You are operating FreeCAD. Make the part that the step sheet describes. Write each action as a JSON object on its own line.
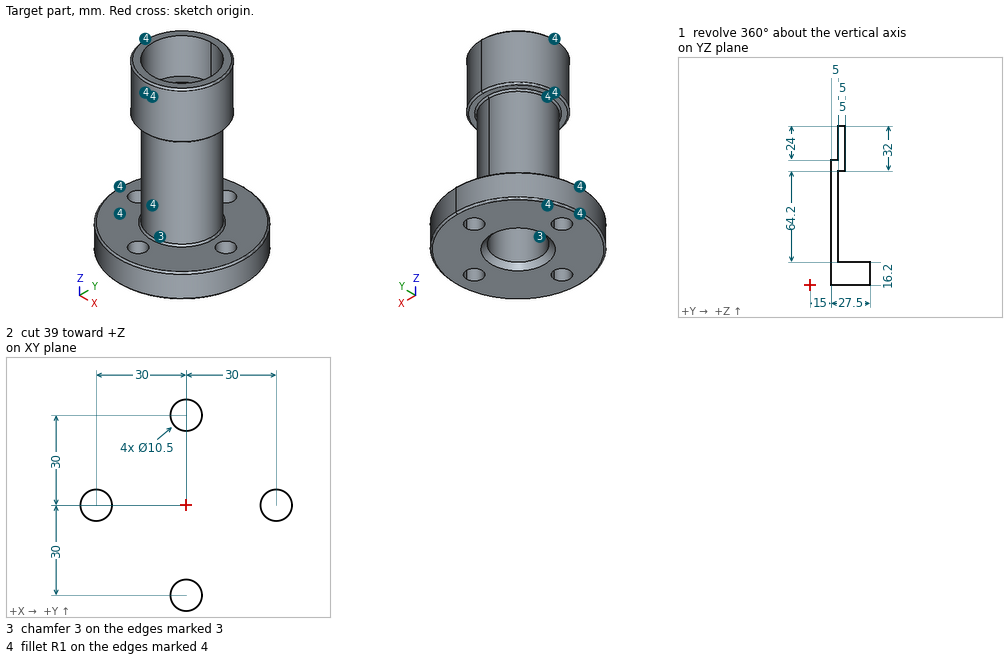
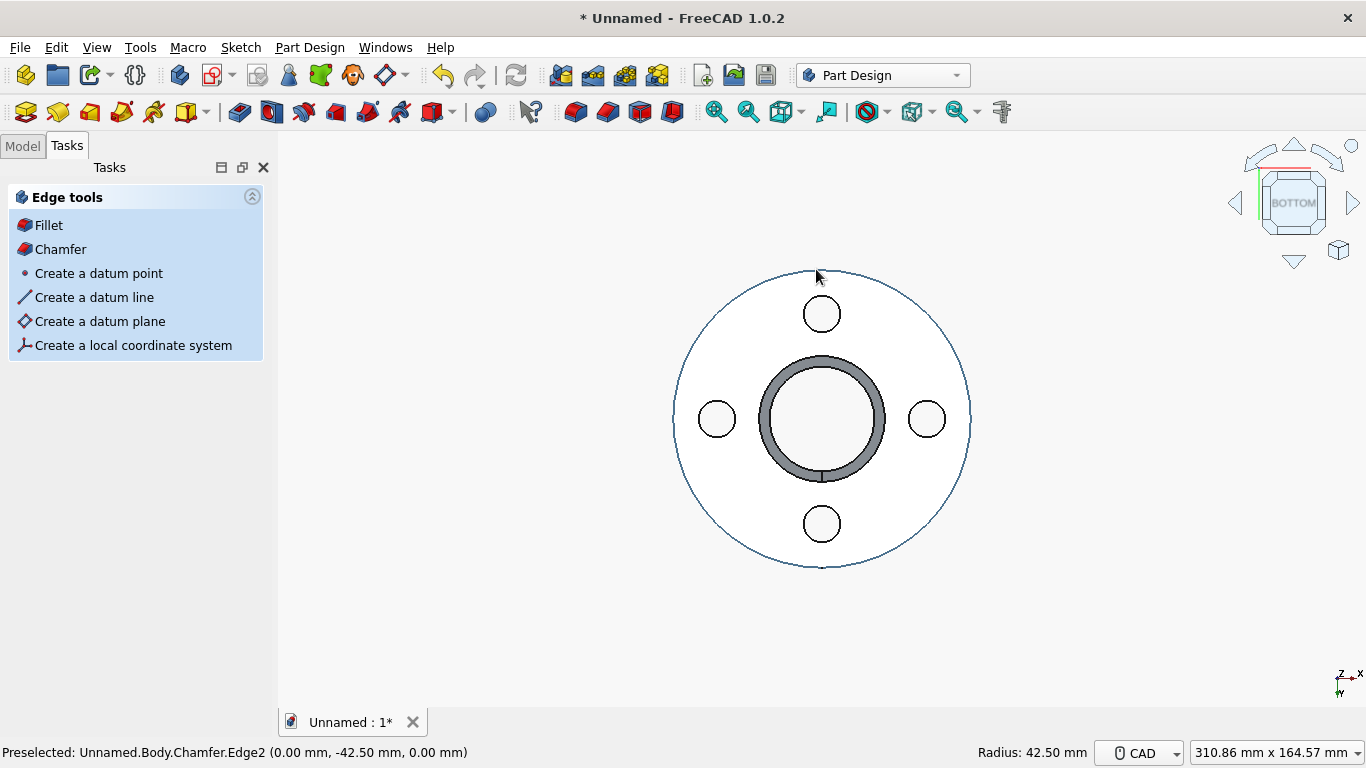
{"action": "key", "text": "0"}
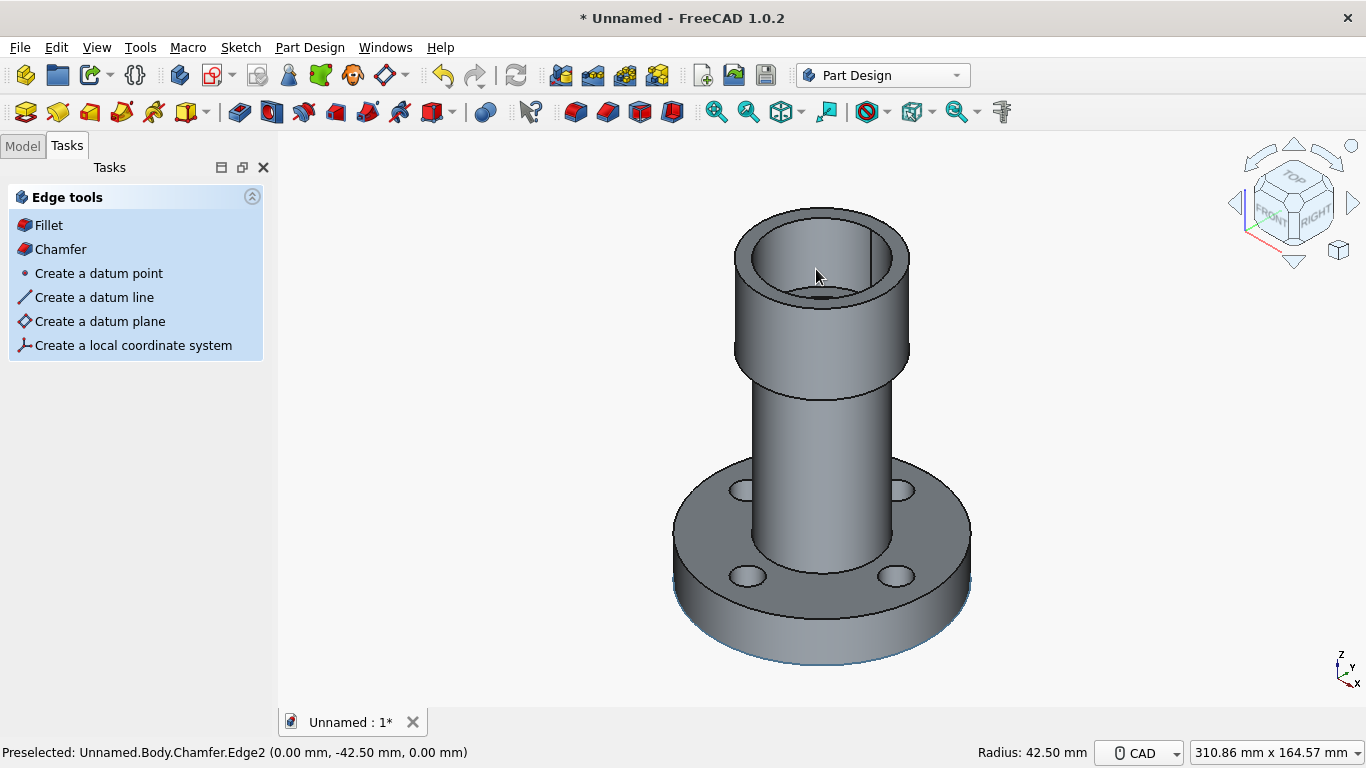
{"action": "left_click", "coordinate": [717, 593], "text": "ctrl"}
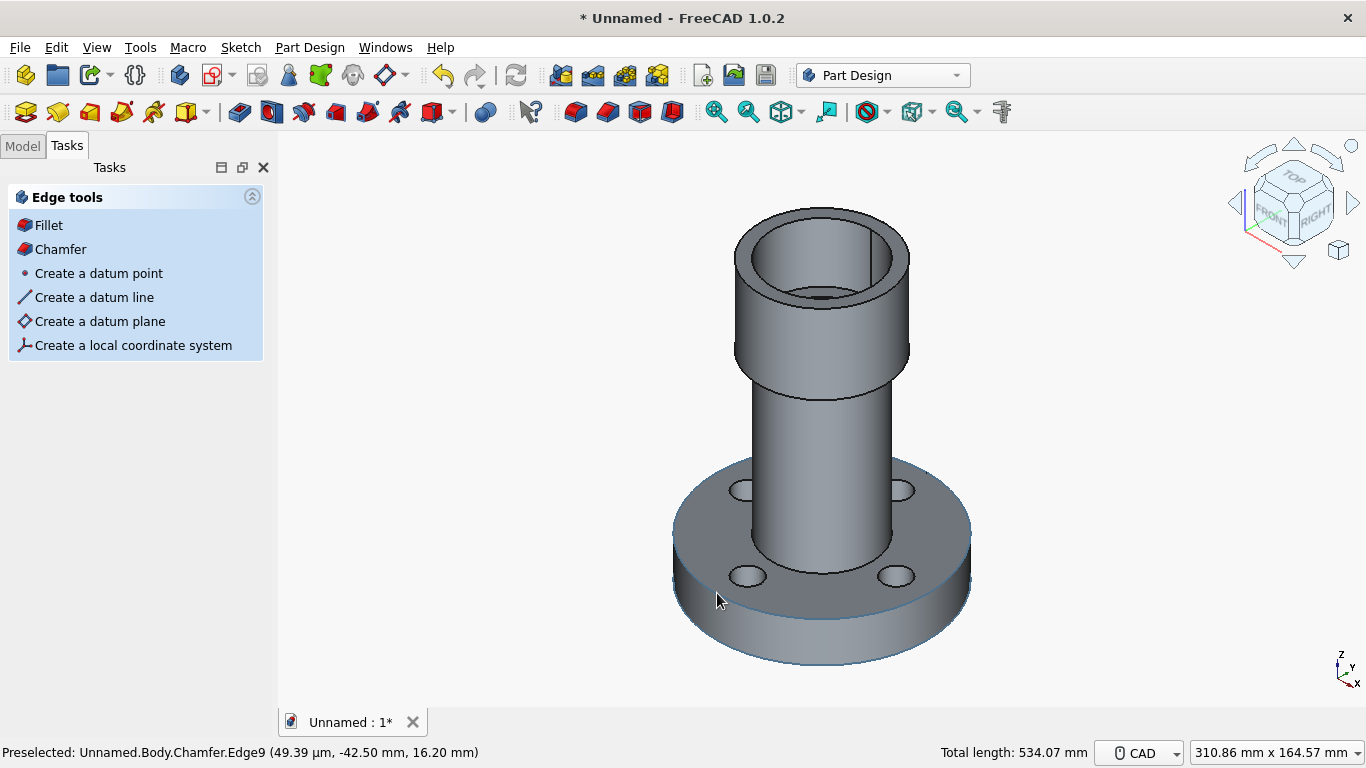
{"action": "left_click", "coordinate": [760, 293], "text": "ctrl"}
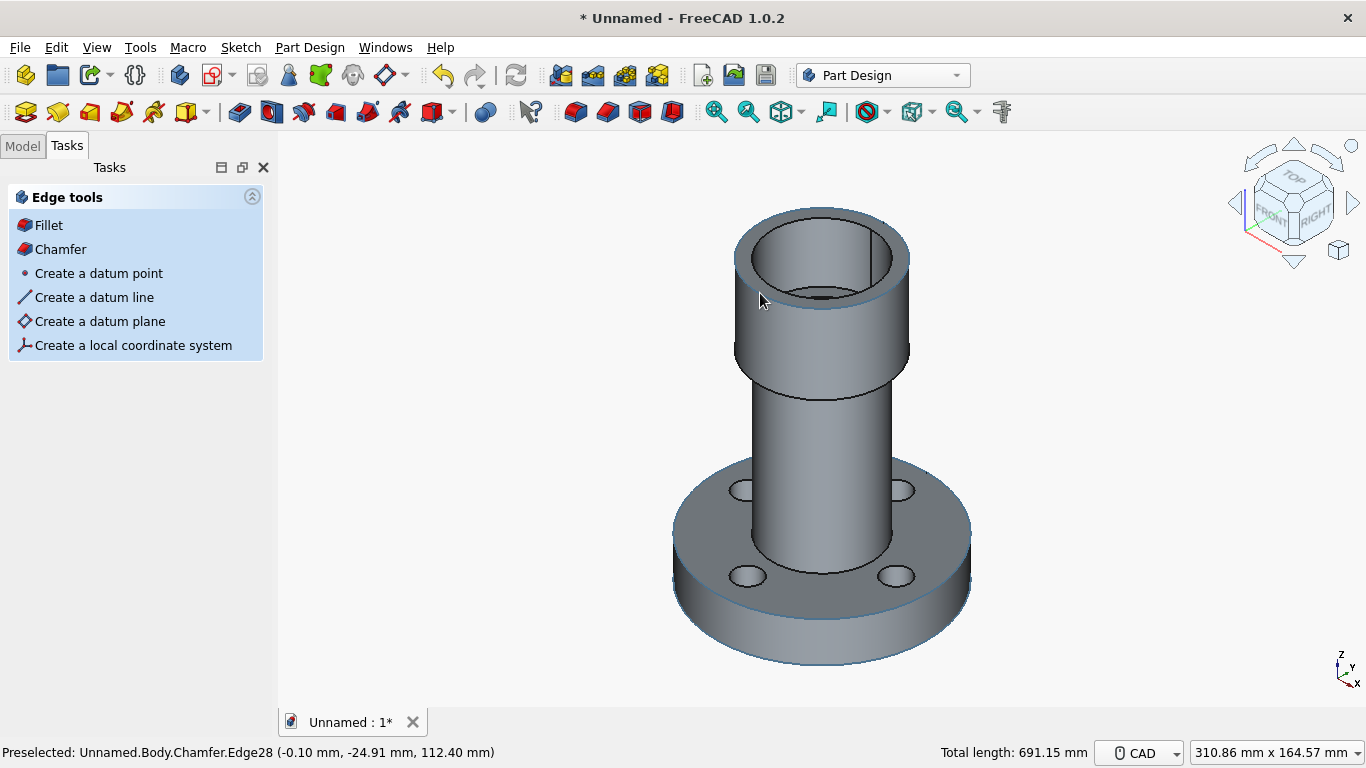
{"action": "key", "text": "2"}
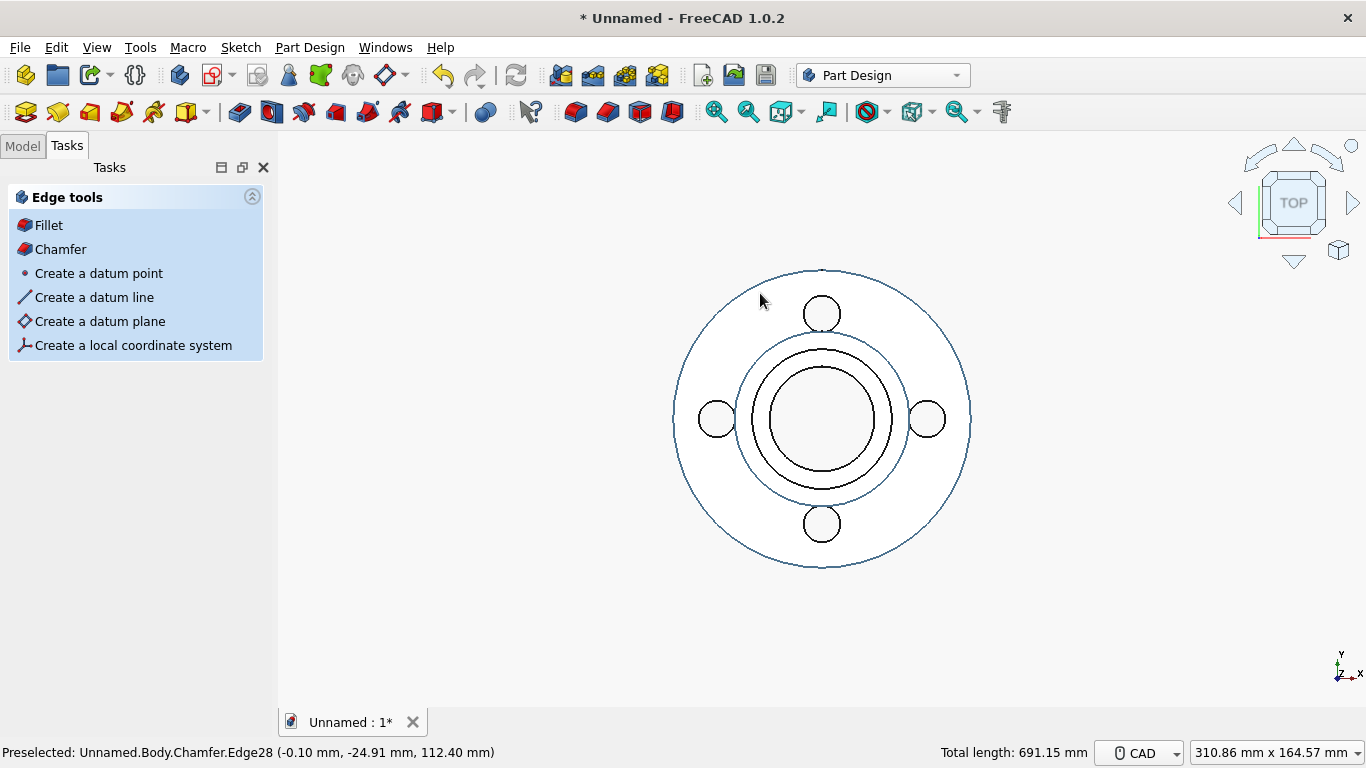
{"action": "key", "text": "1"}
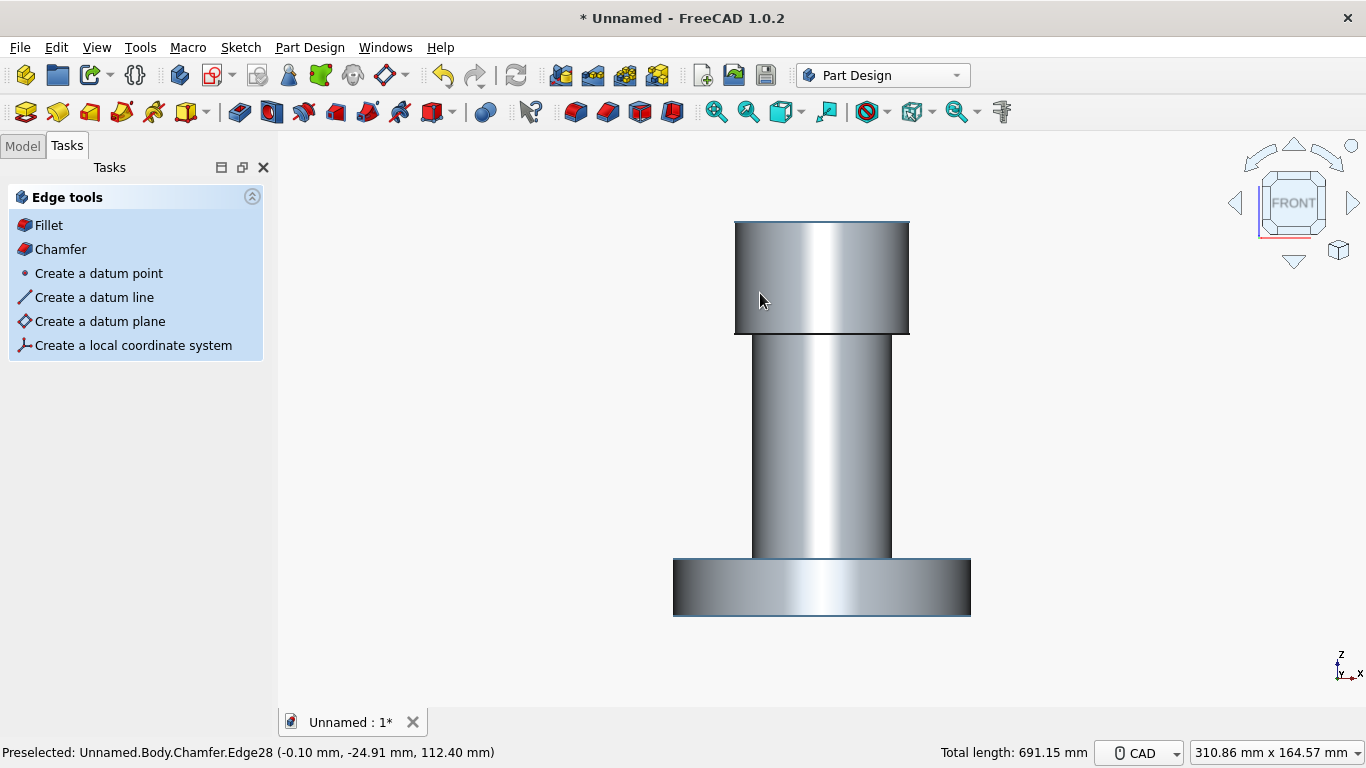
{"action": "left_click", "coordinate": [822, 333], "text": "ctrl"}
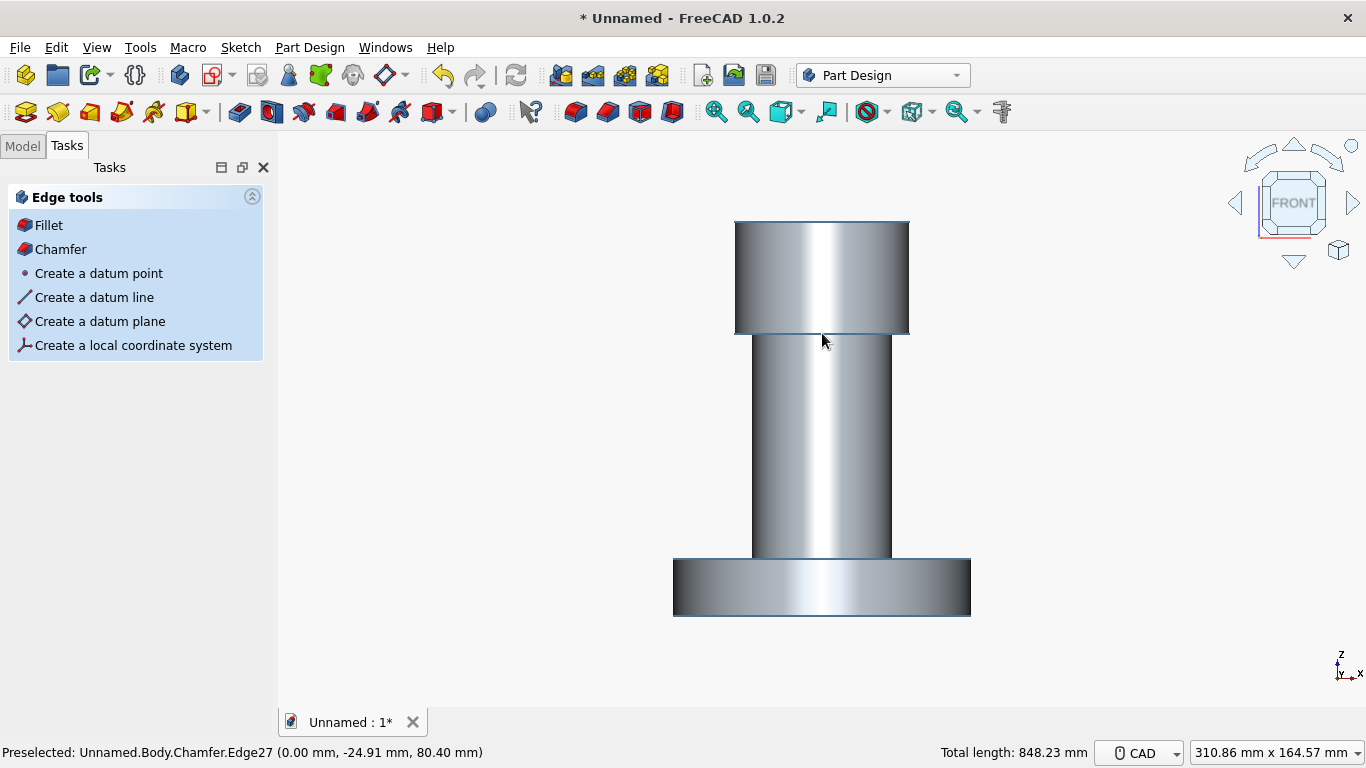
{"action": "key", "text": "3"}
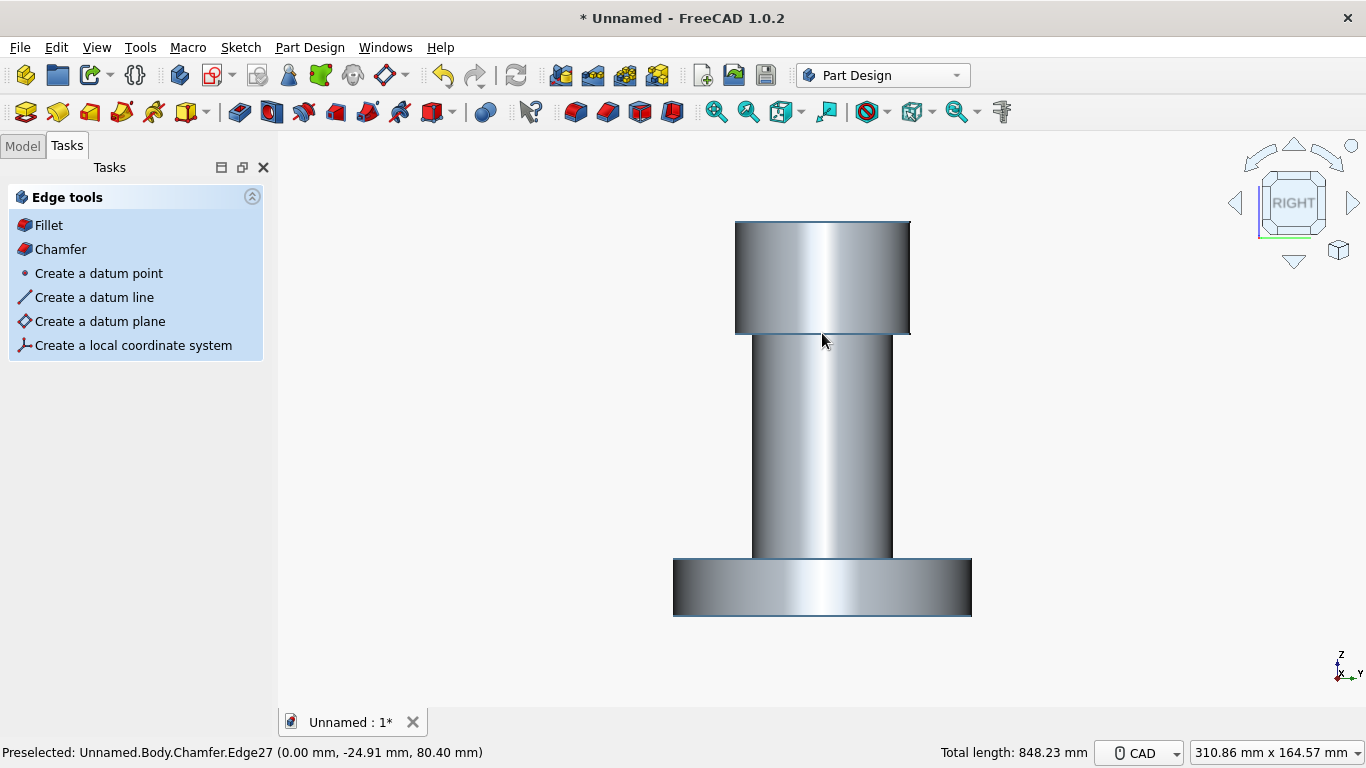
{"action": "key", "text": "5"}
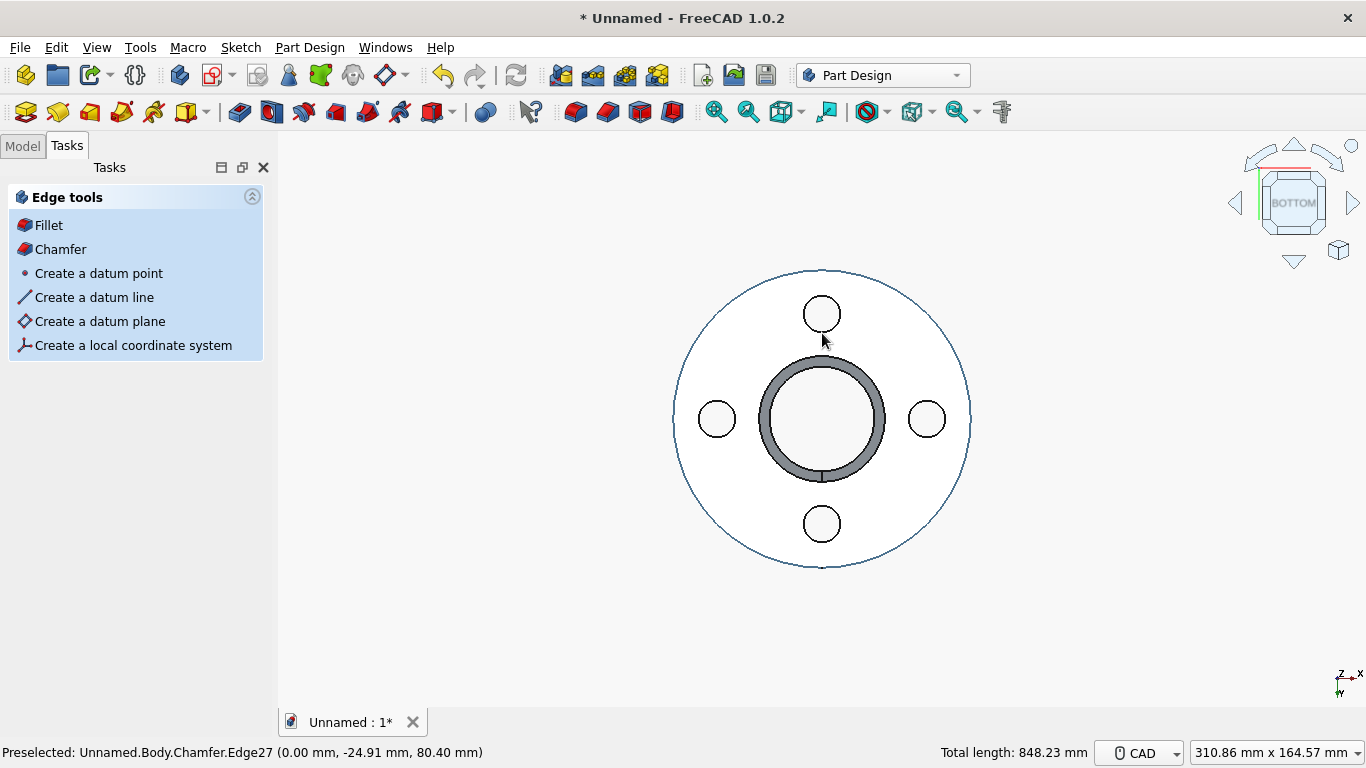
{"action": "key", "text": "4"}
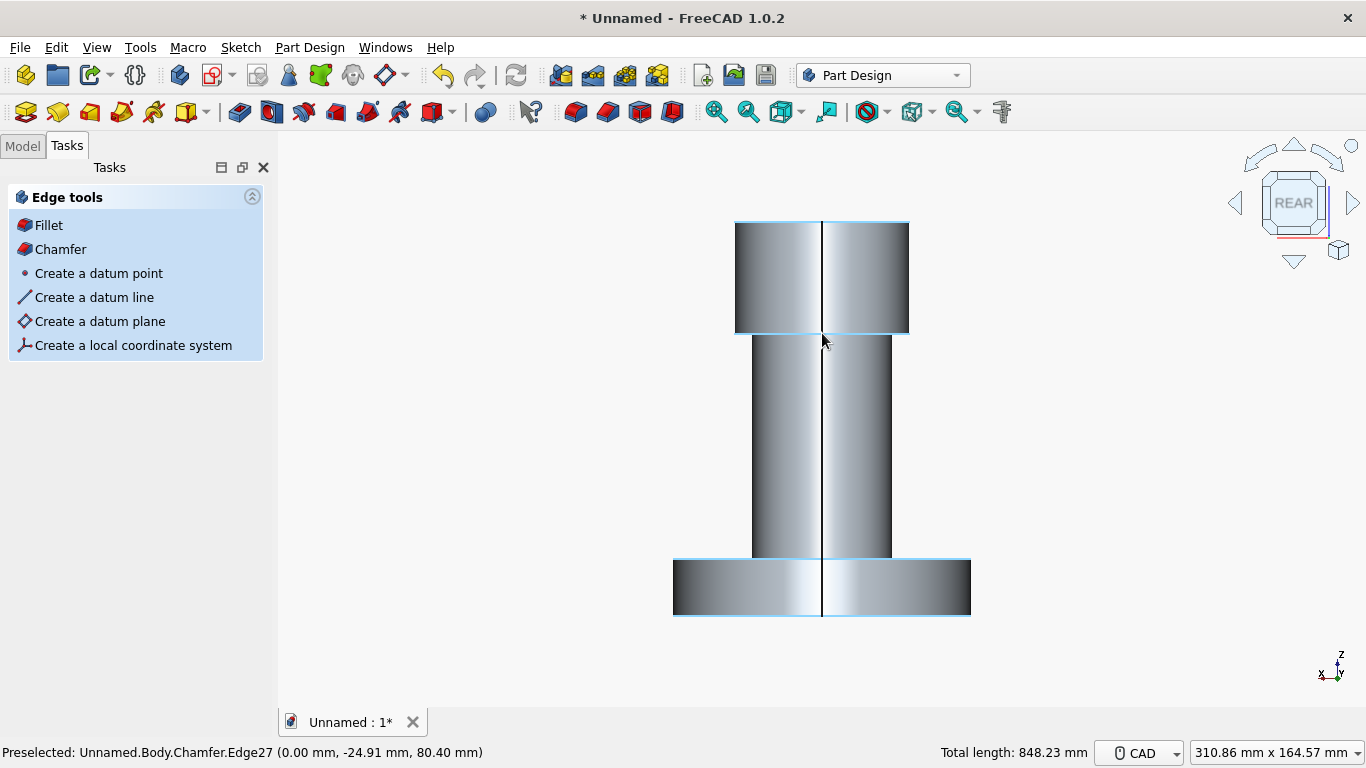
{"action": "key", "text": "6"}